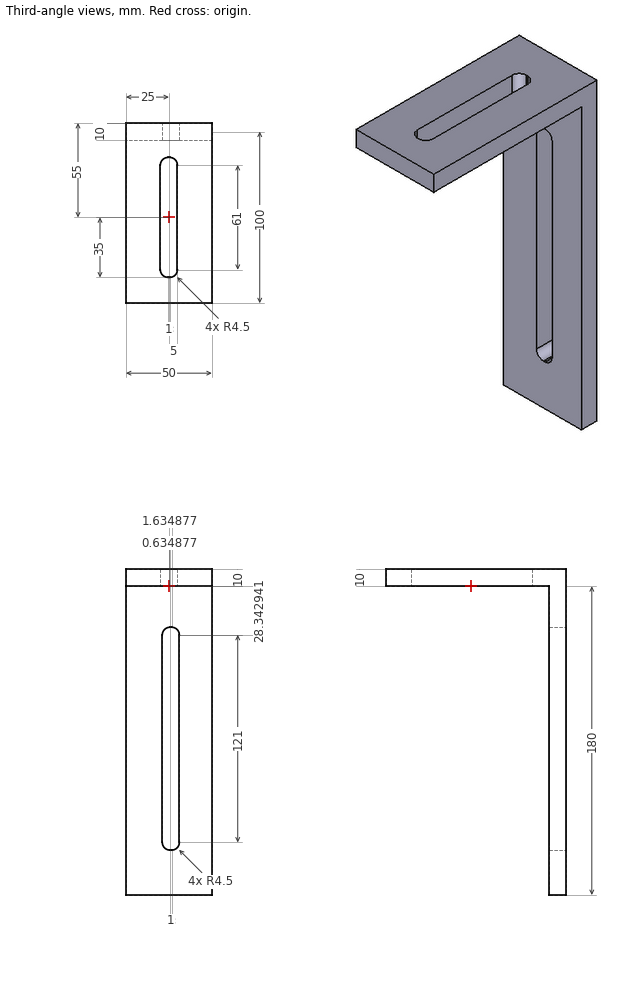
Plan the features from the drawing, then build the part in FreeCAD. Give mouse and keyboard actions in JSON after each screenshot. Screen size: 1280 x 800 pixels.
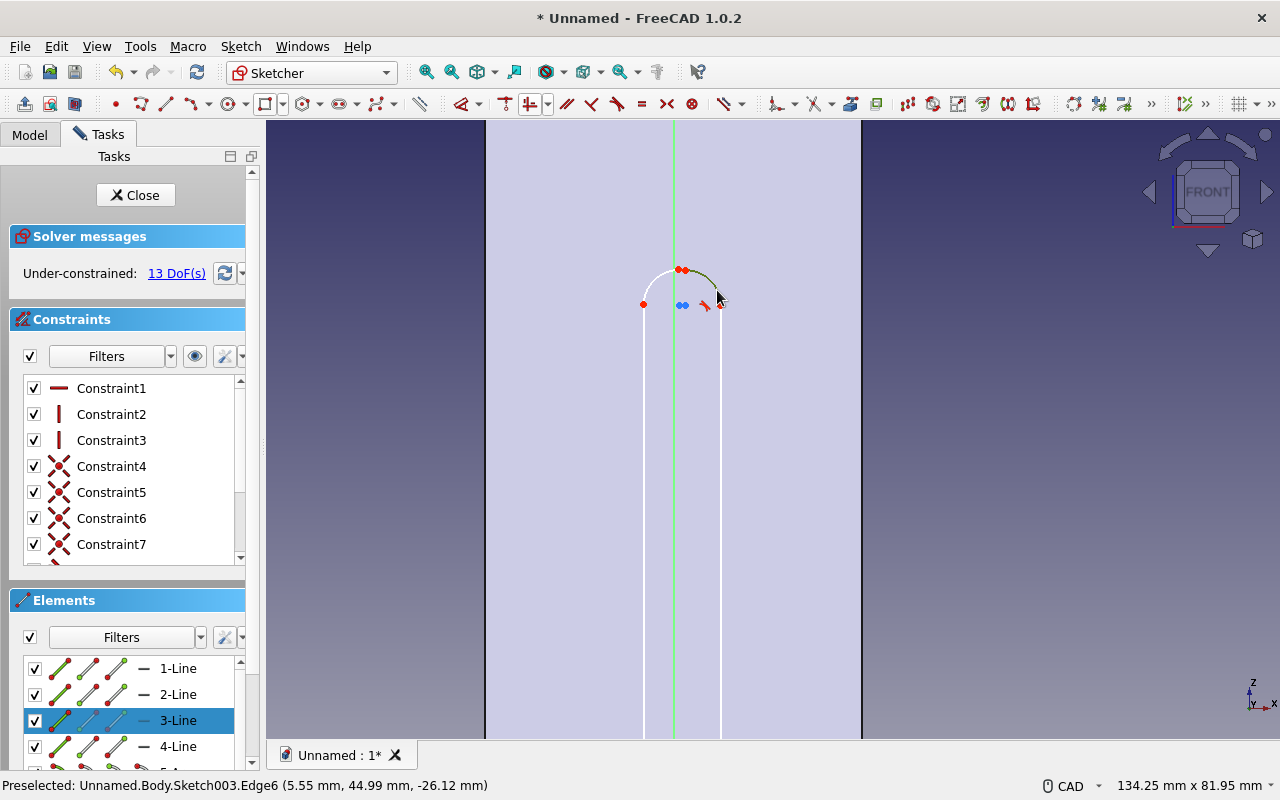
{"action": "left_click", "coordinate": [617, 104]}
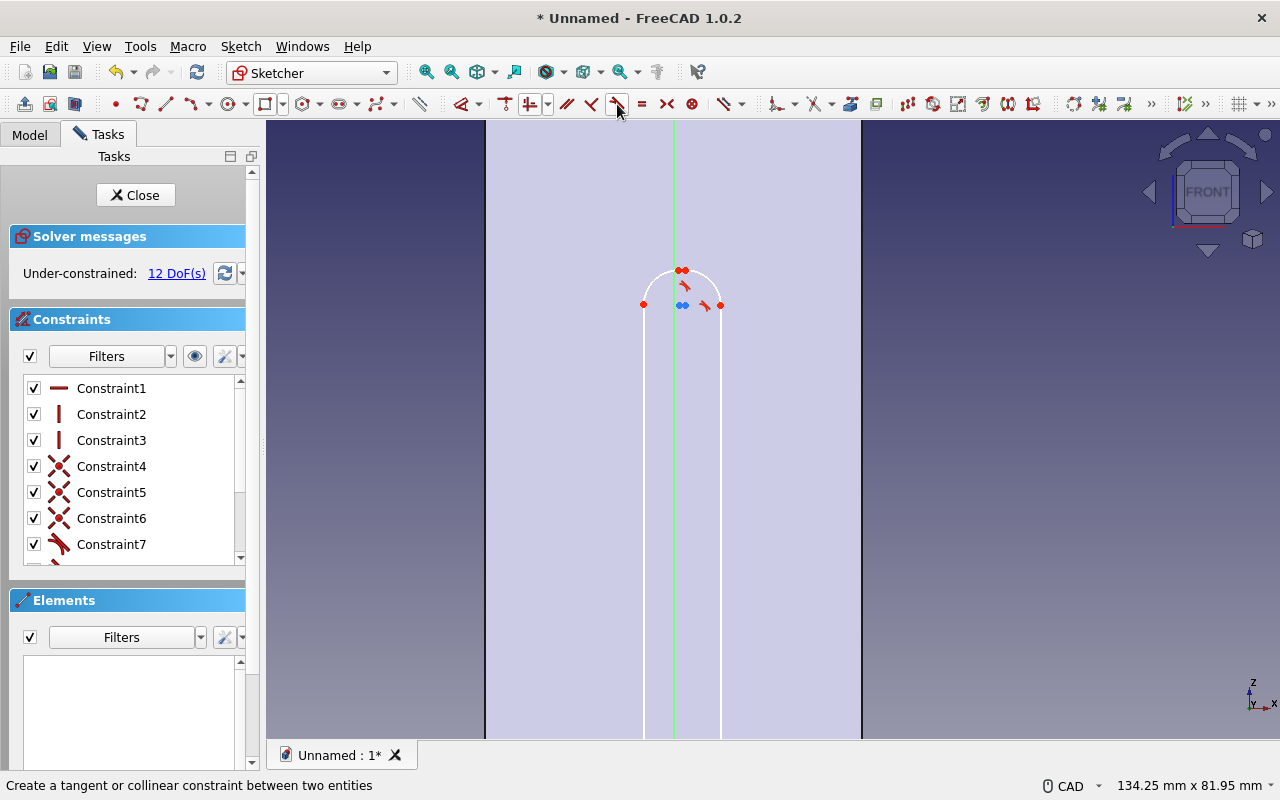
{"action": "scroll", "coordinate": [682, 270], "scroll_direction": "up", "scroll_amount": 7}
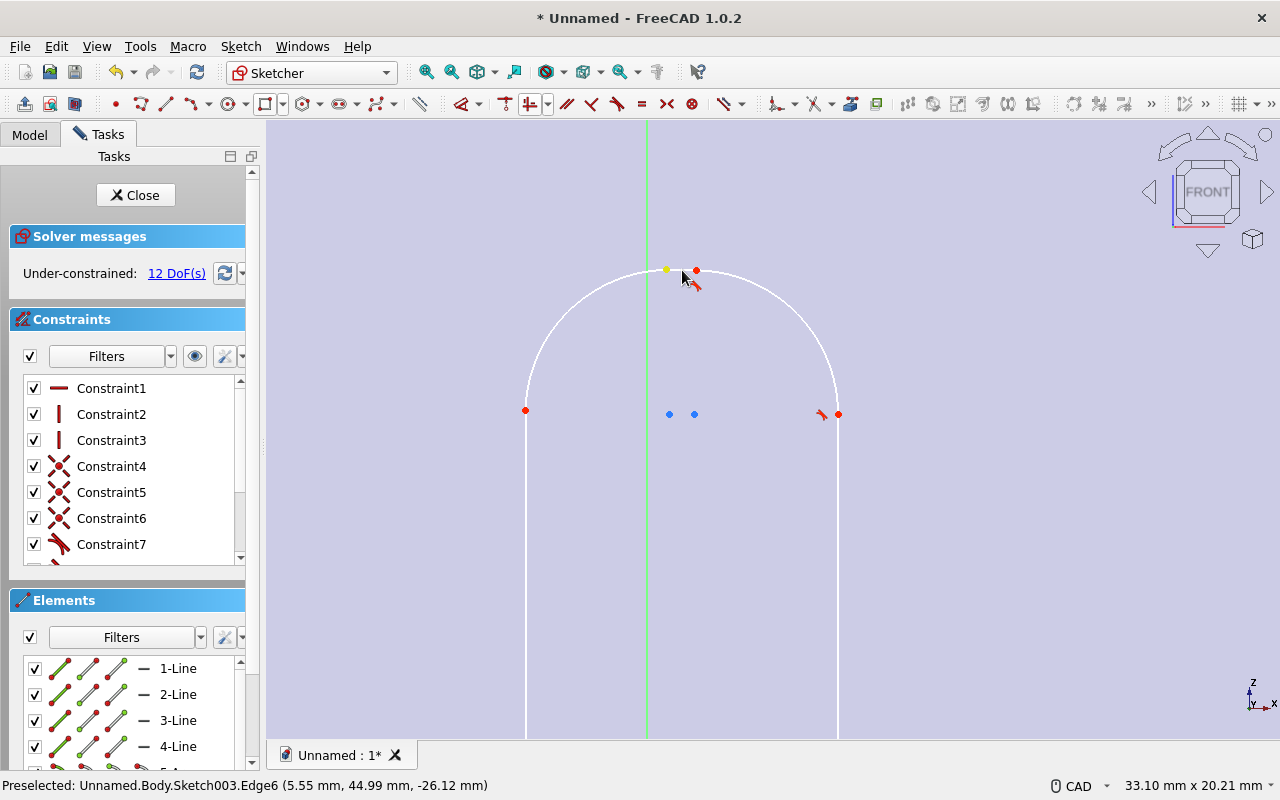
{"action": "left_click", "coordinate": [681, 270]}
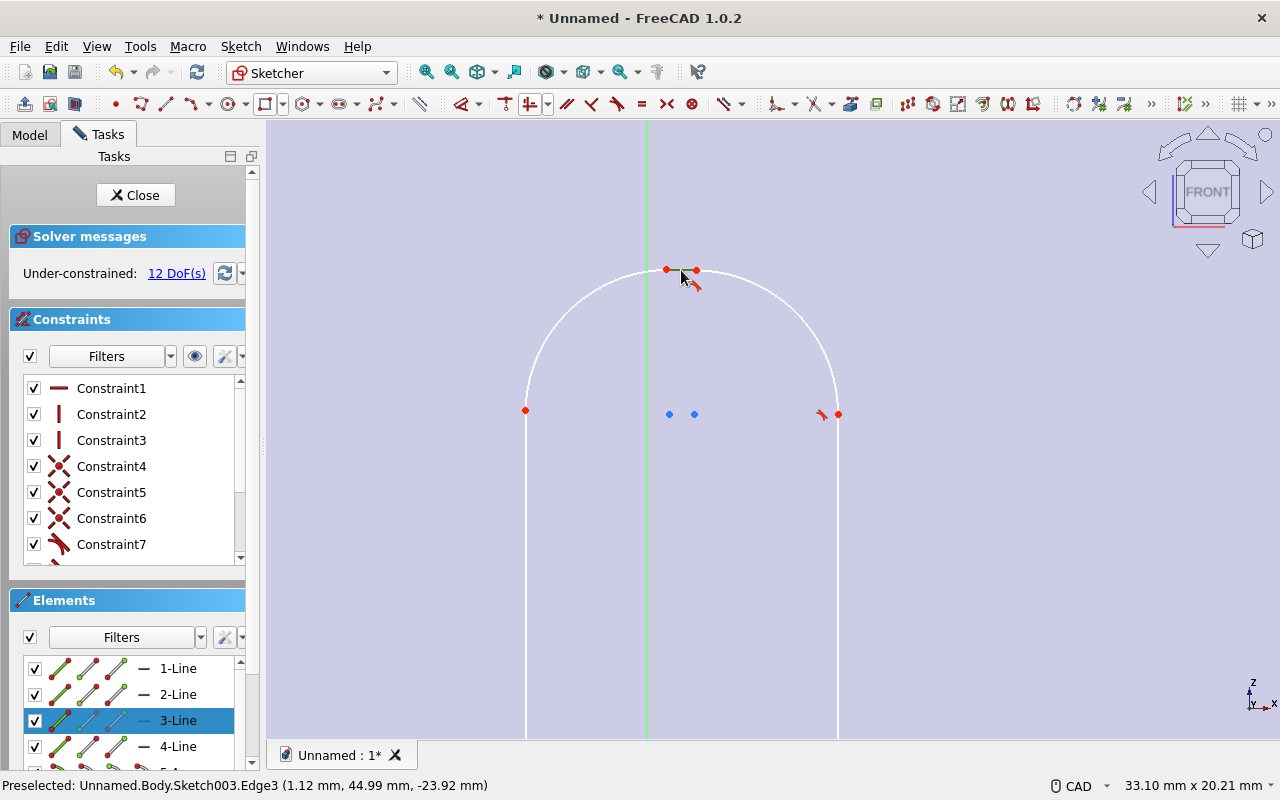
{"action": "scroll", "coordinate": [707, 283], "scroll_direction": "down", "scroll_amount": 12}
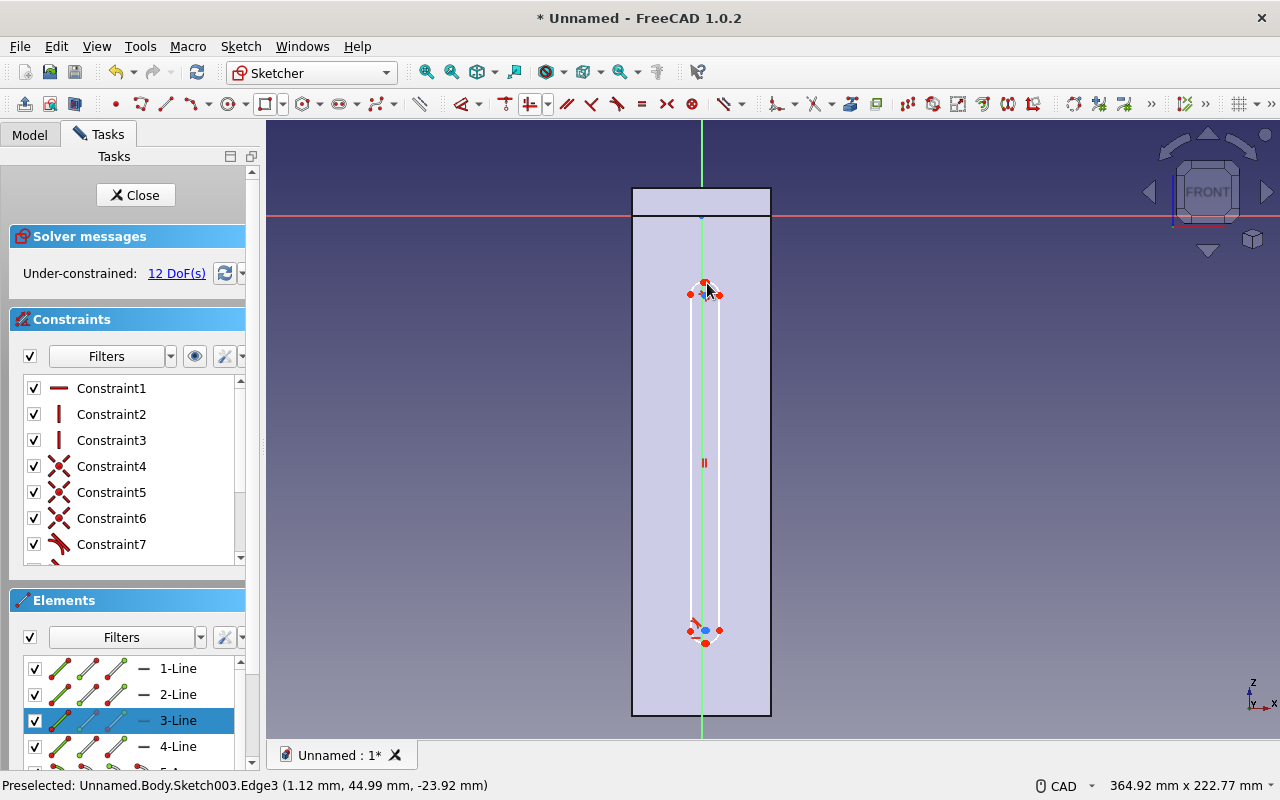
{"action": "scroll", "coordinate": [698, 284], "scroll_direction": "up", "scroll_amount": 7}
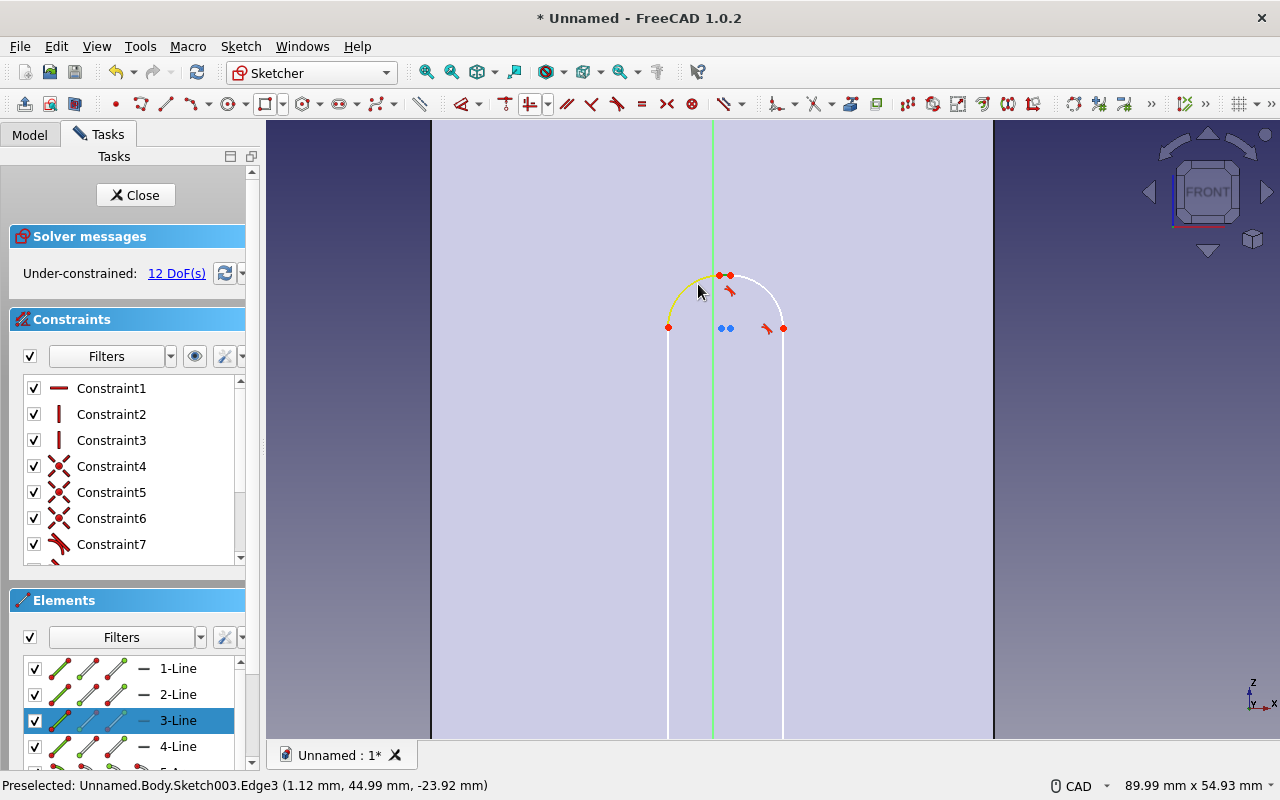
{"action": "left_click", "coordinate": [696, 281]}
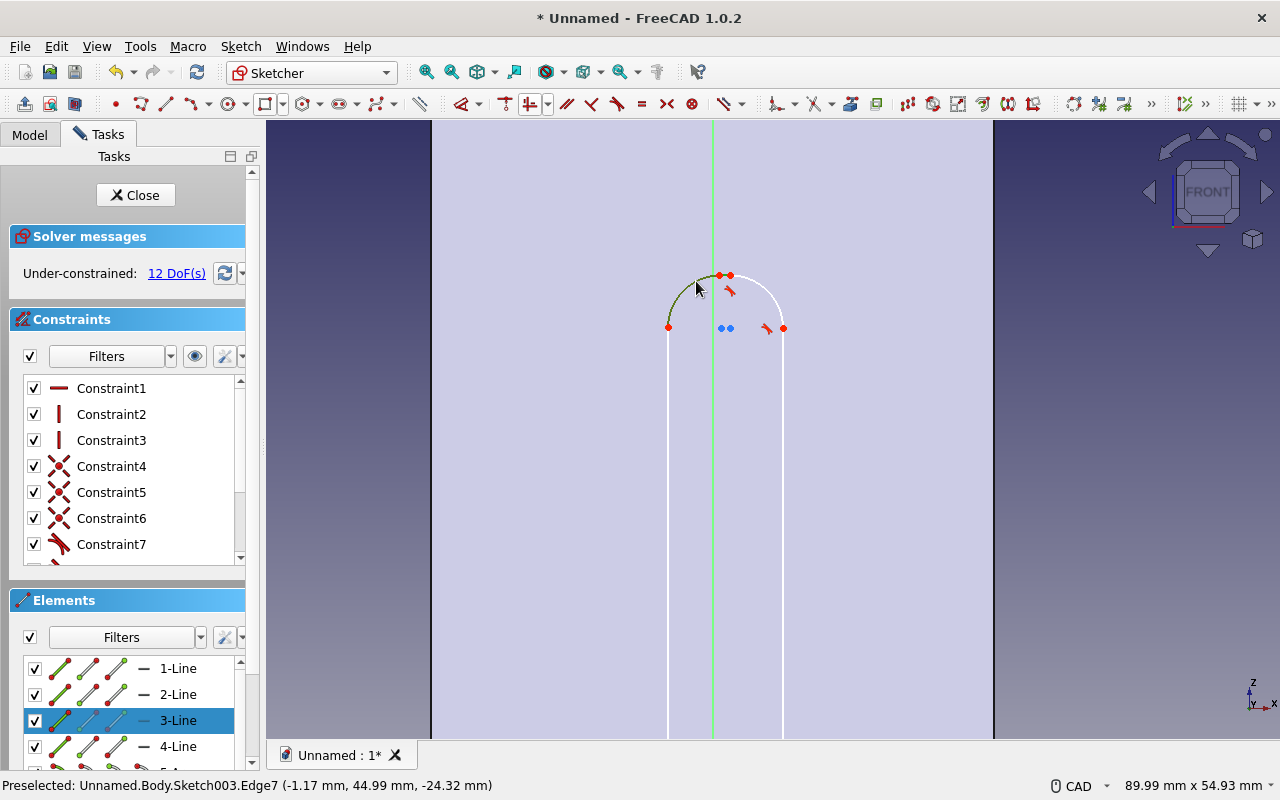
{"action": "left_click", "coordinate": [617, 104]}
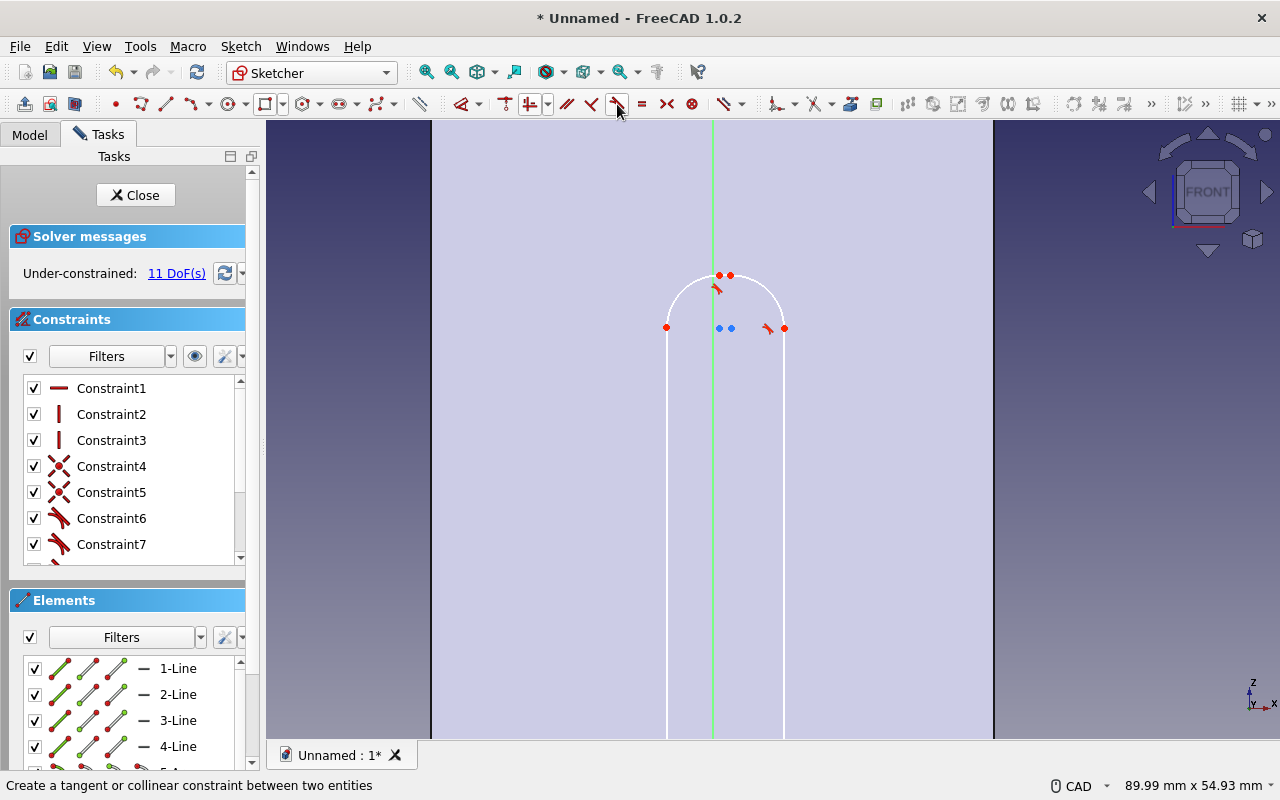
{"action": "scroll", "coordinate": [698, 284], "scroll_direction": "down", "scroll_amount": 7}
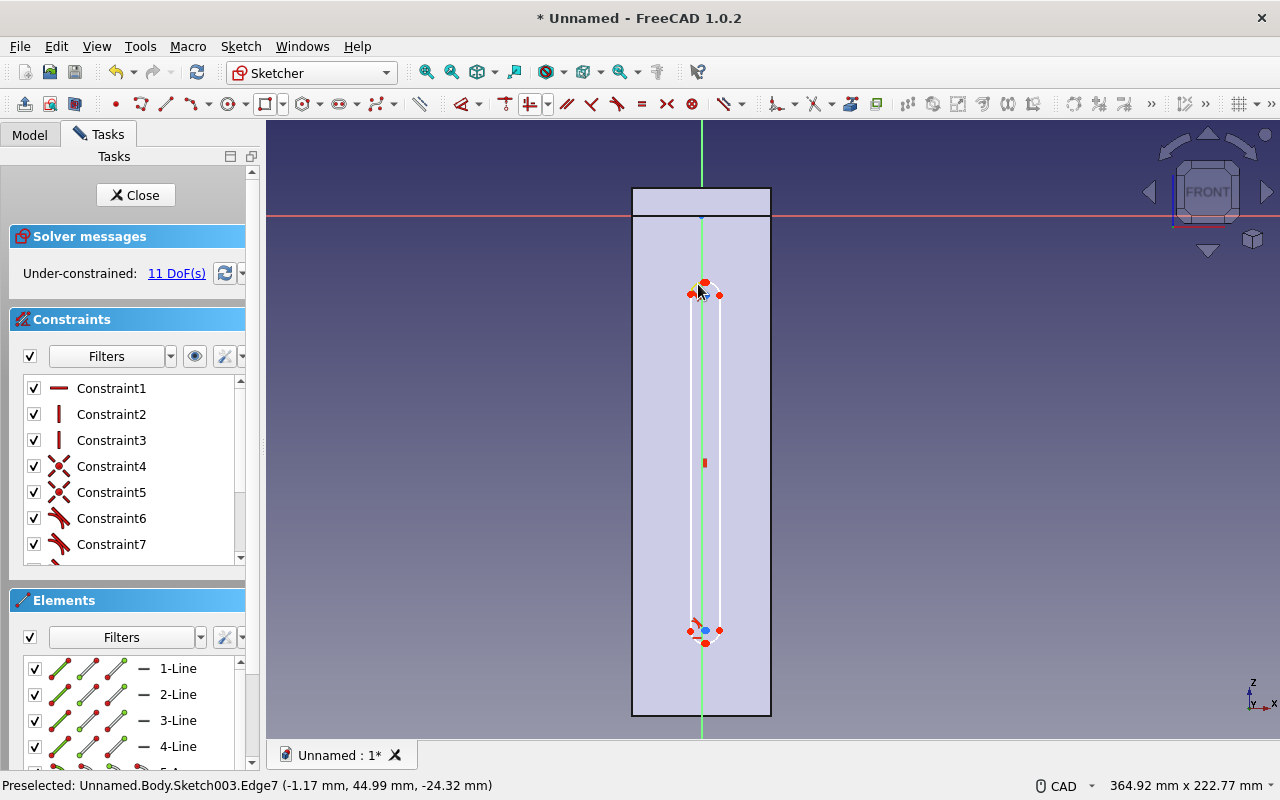
{"action": "scroll", "coordinate": [691, 362], "scroll_direction": "up", "scroll_amount": 2}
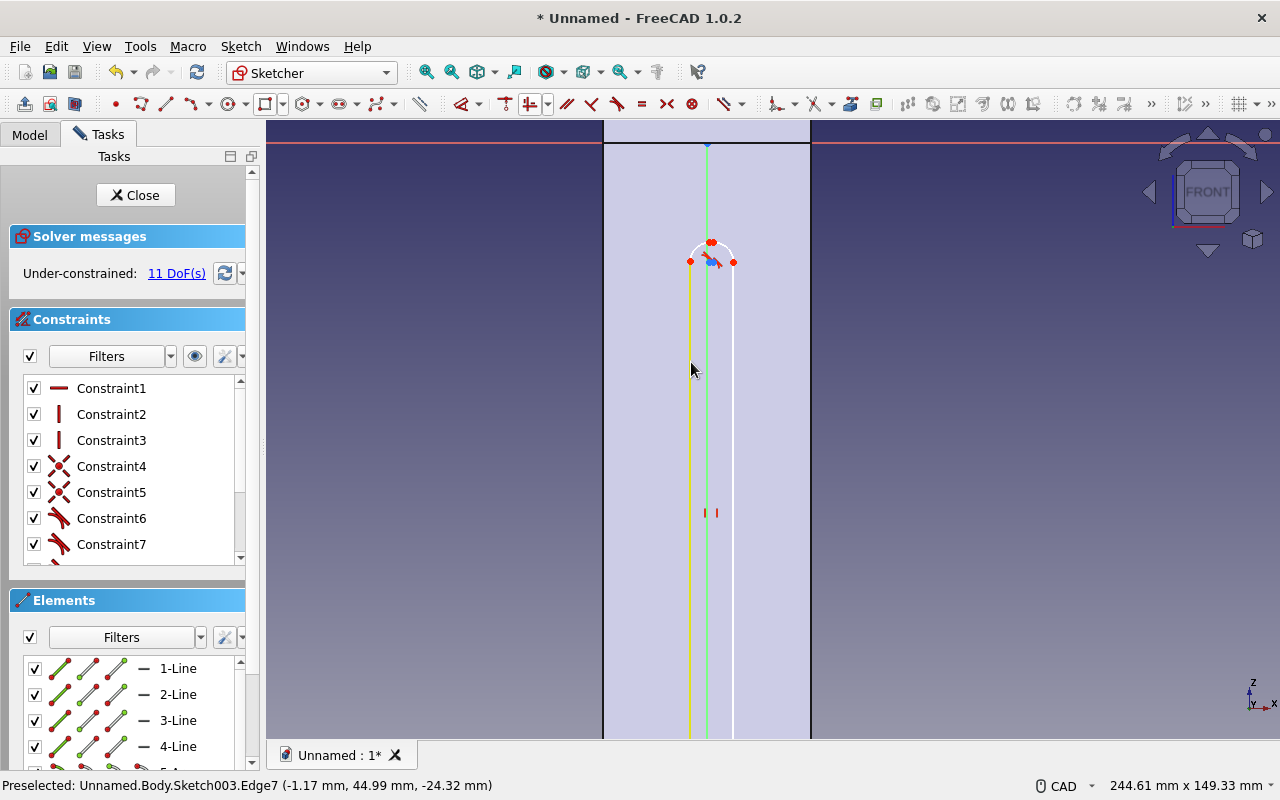
{"action": "left_click", "coordinate": [690, 362]}